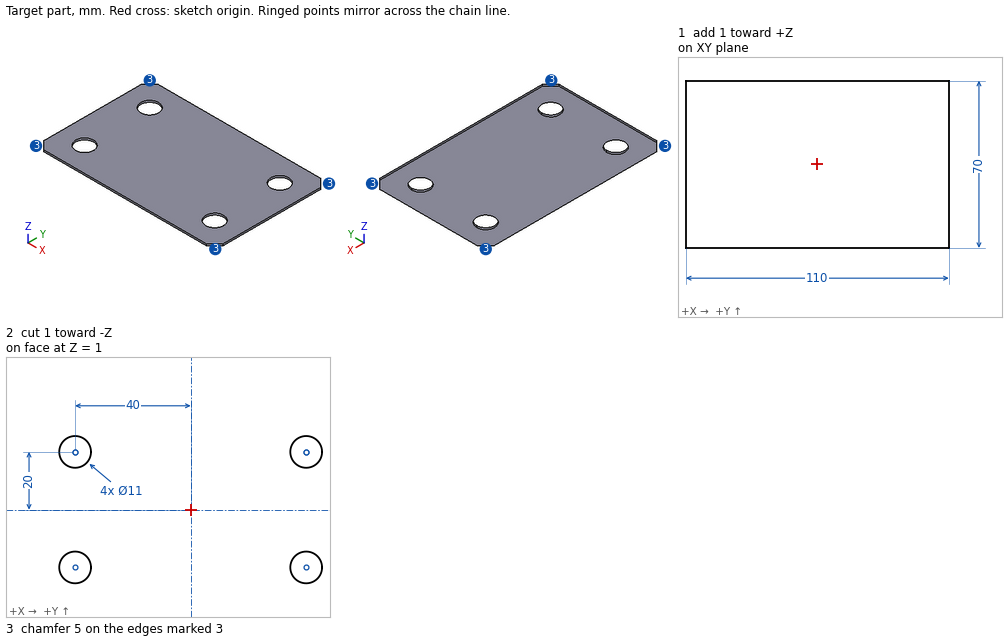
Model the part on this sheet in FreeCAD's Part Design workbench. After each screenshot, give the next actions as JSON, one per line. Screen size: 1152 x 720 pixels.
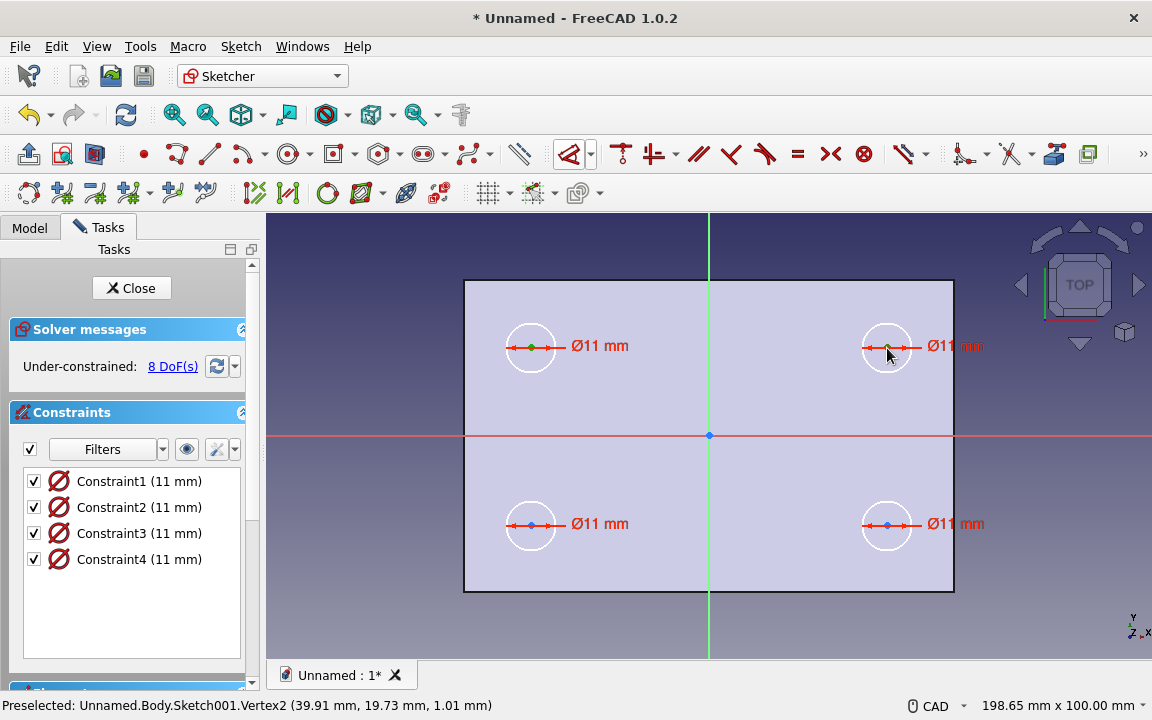
{"action": "left_click", "coordinate": [709, 603]}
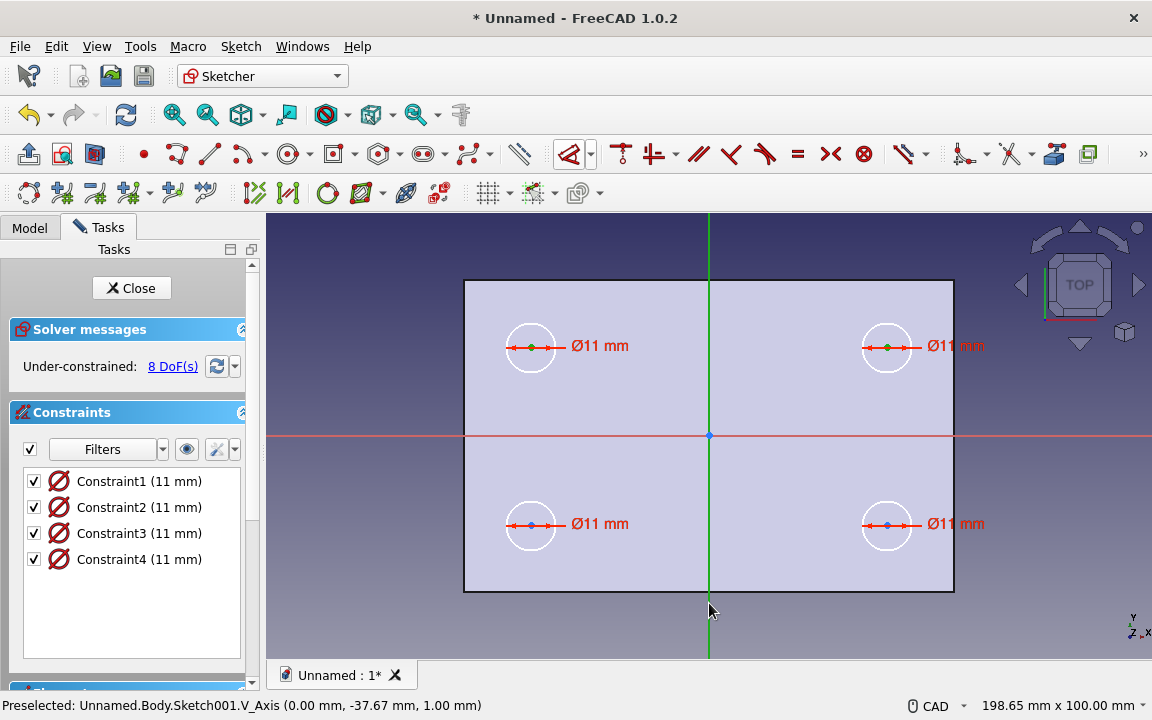
{"action": "left_click", "coordinate": [831, 154]}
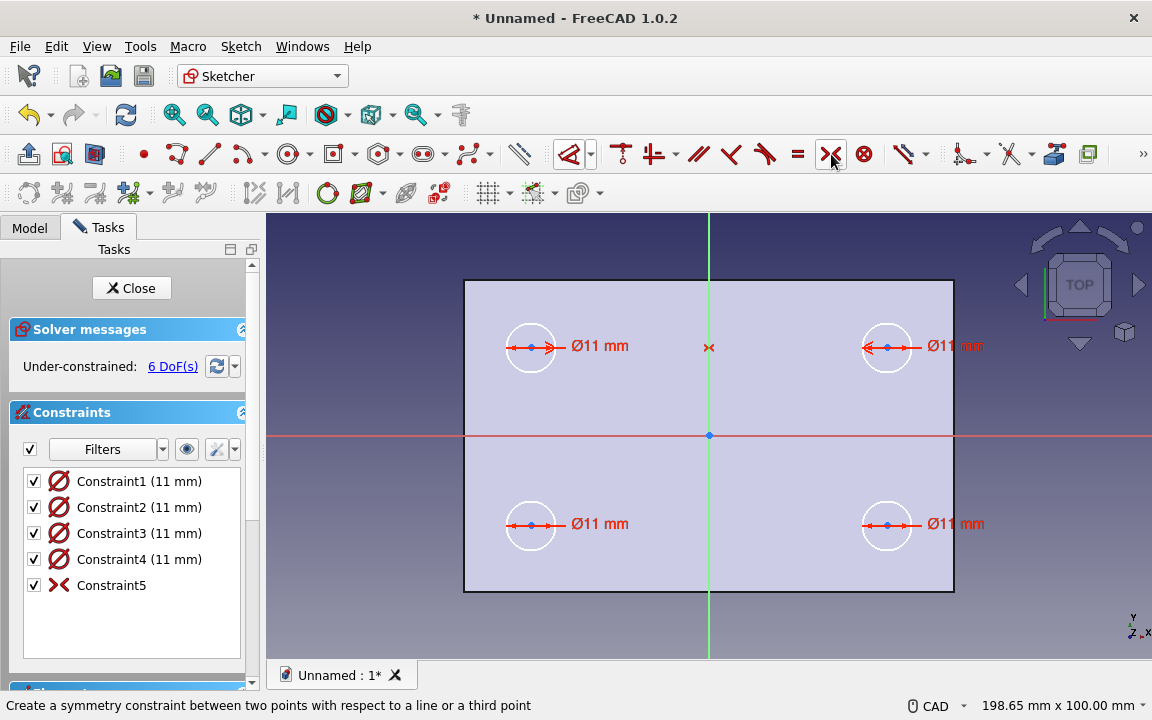
{"action": "left_click", "coordinate": [531, 348]}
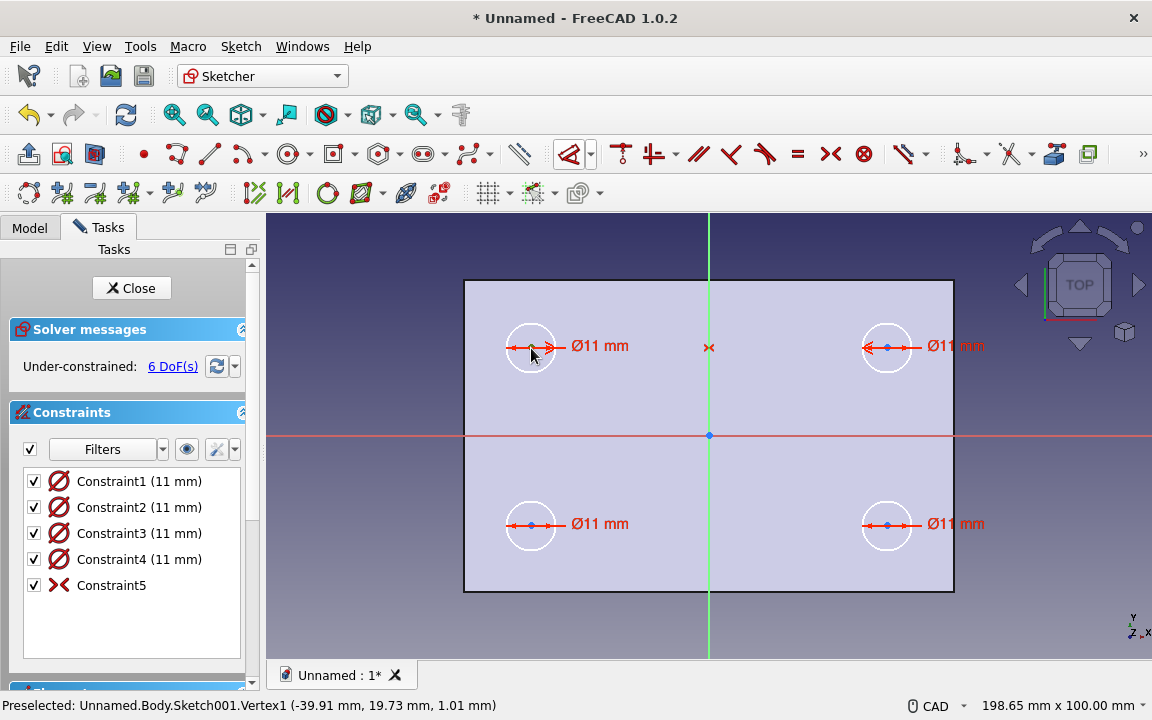
{"action": "left_click", "coordinate": [531, 526]}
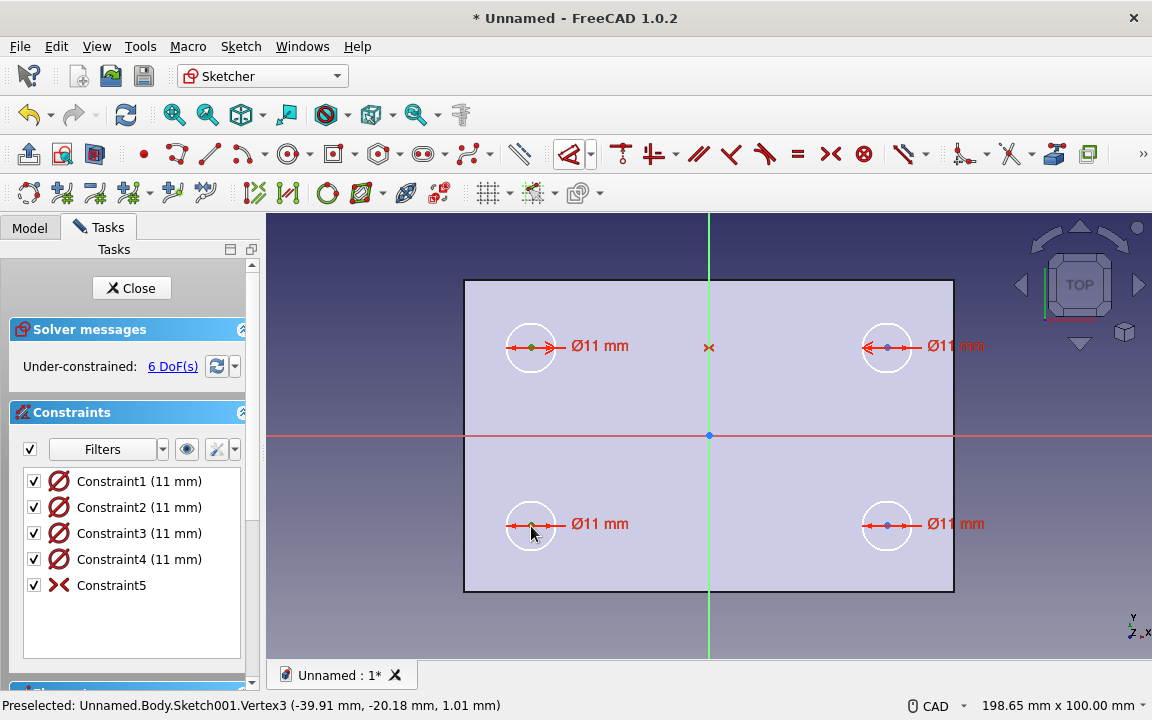
{"action": "left_click", "coordinate": [344, 436]}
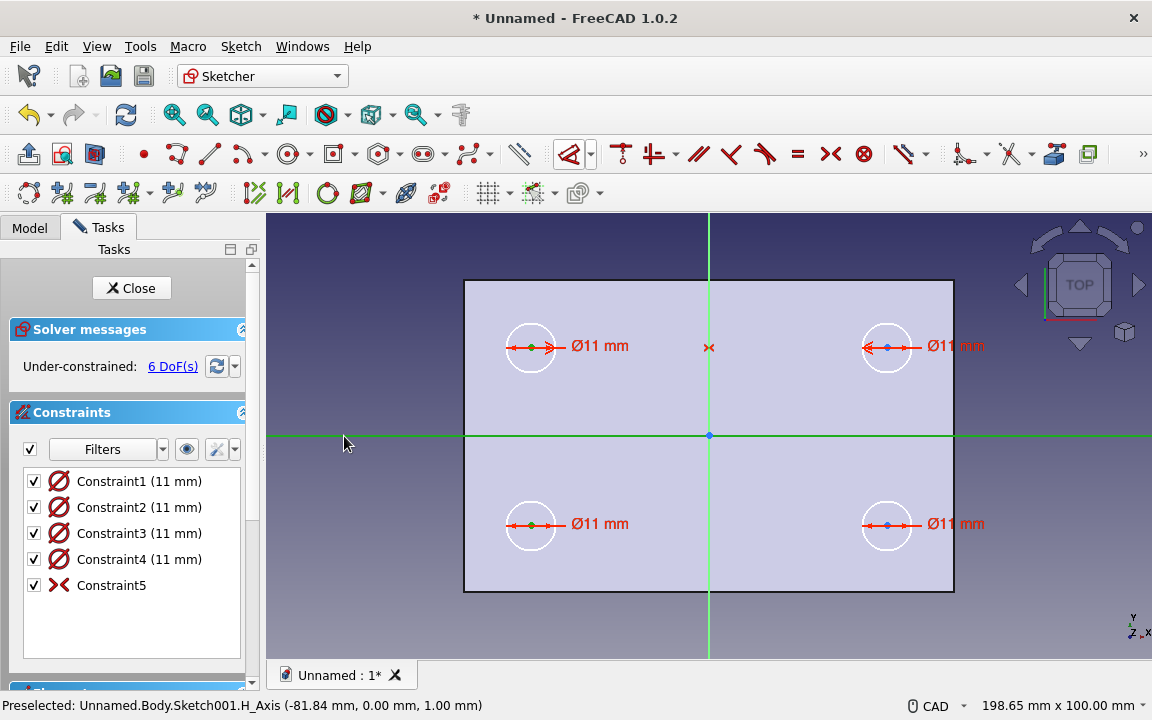
{"action": "left_click", "coordinate": [831, 154]}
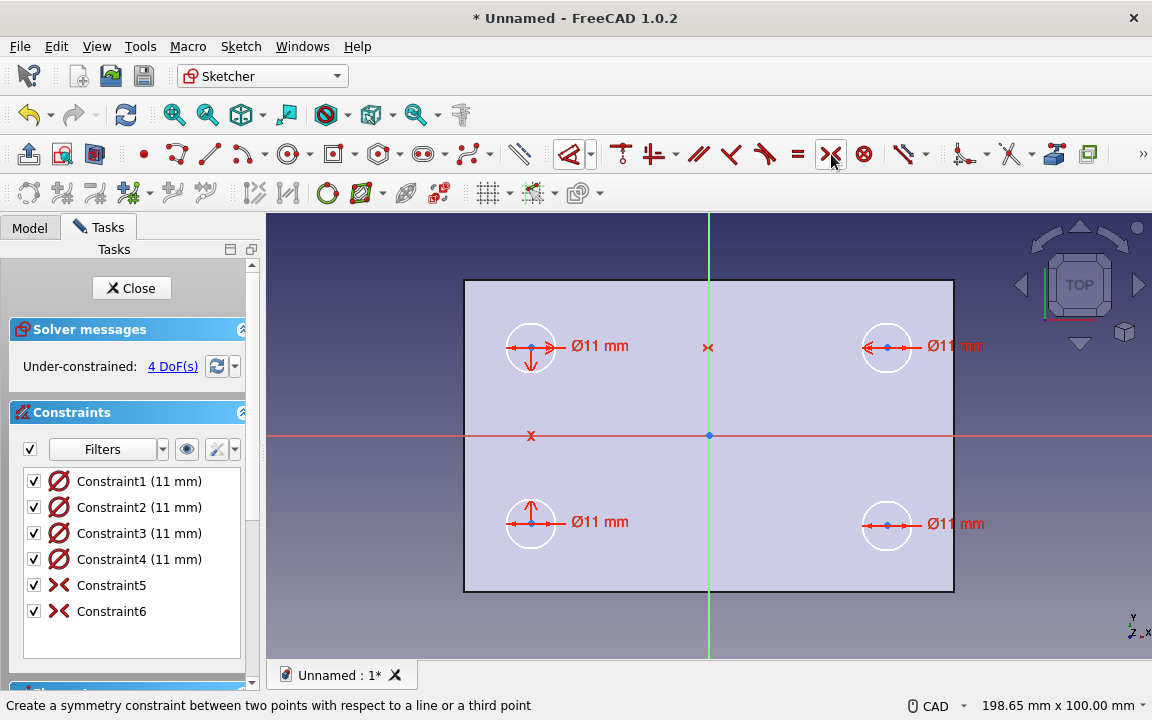
{"action": "left_click", "coordinate": [887, 348]}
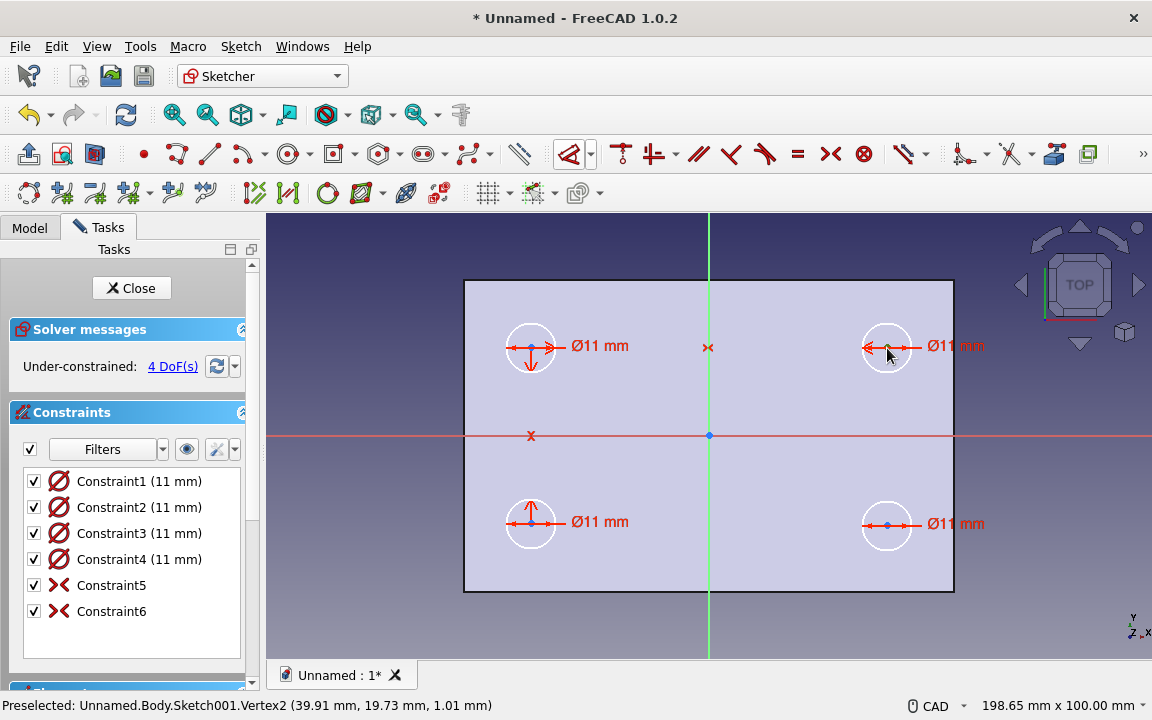
{"action": "left_click", "coordinate": [887, 526]}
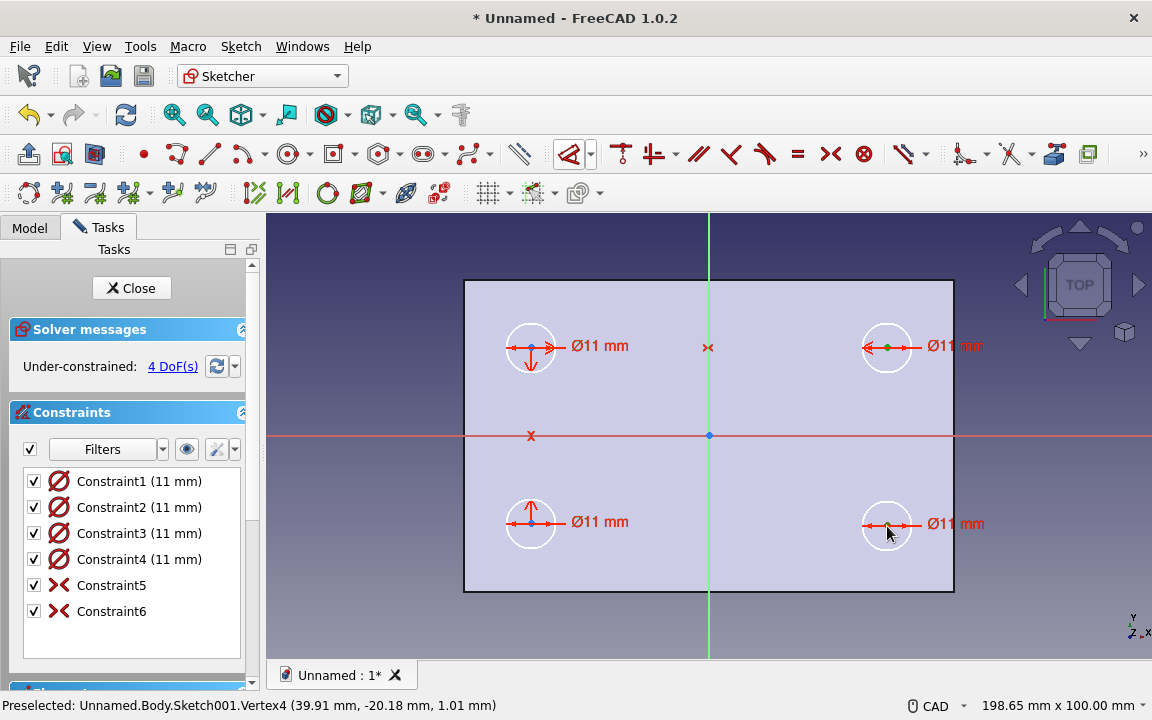
{"action": "left_click", "coordinate": [344, 436]}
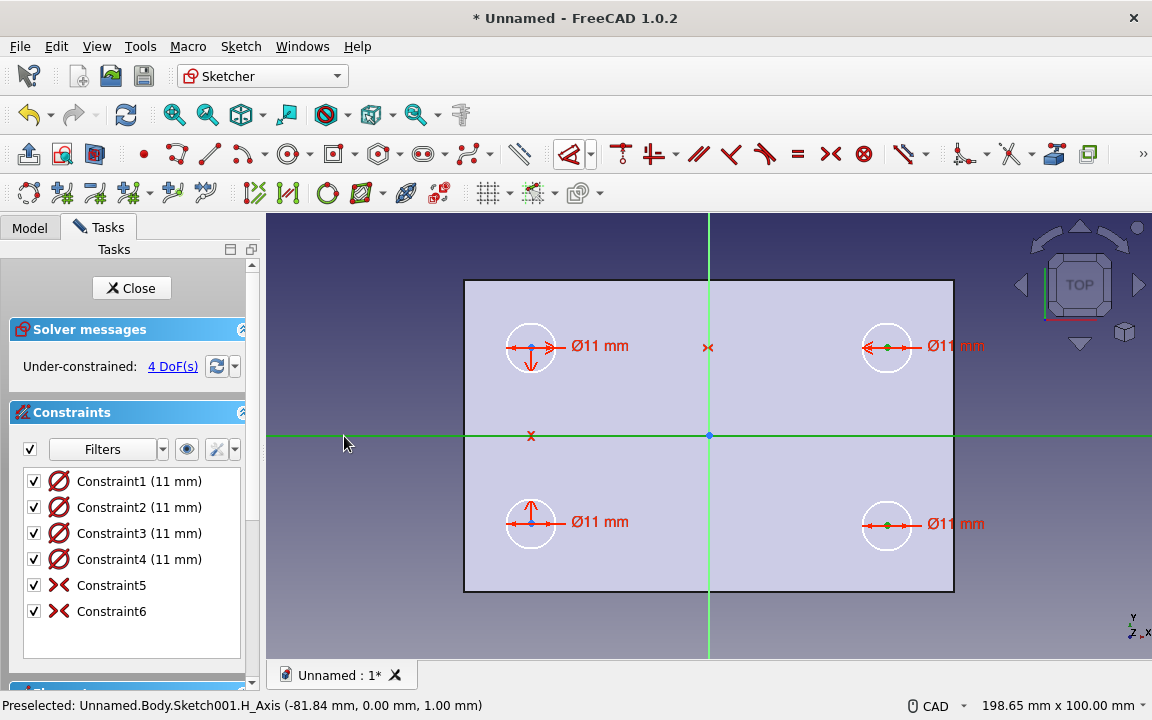
{"action": "left_click", "coordinate": [831, 154]}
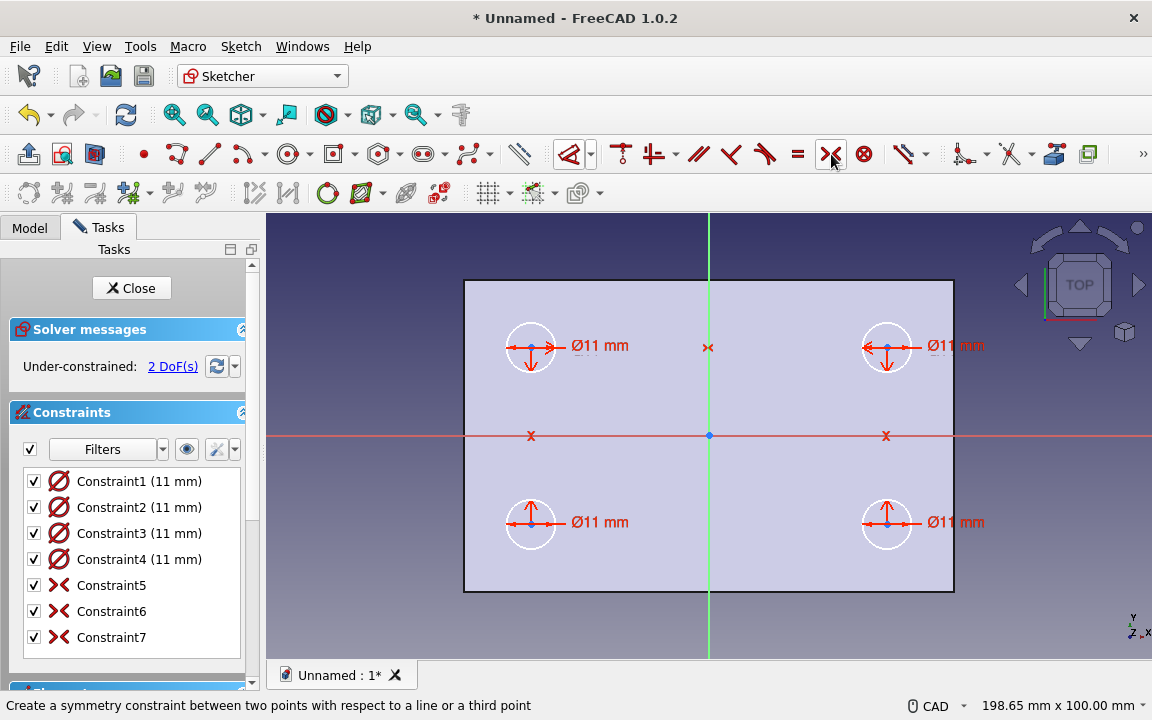
{"action": "left_click", "coordinate": [568, 154]}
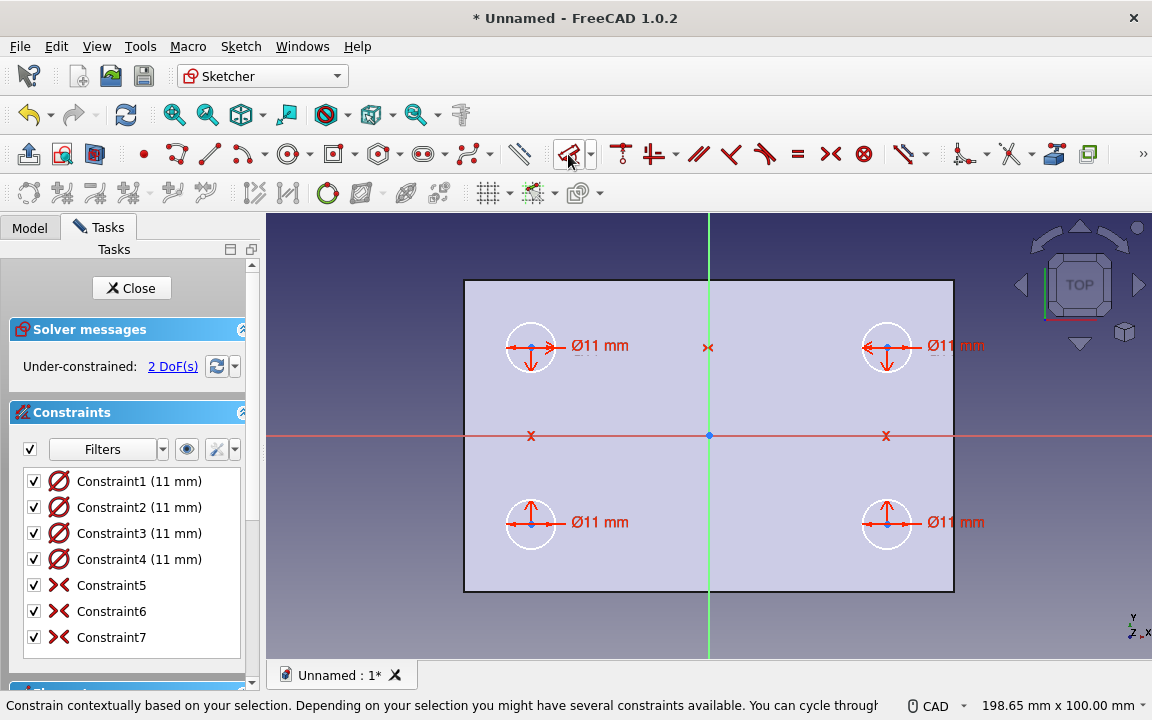
{"action": "left_click", "coordinate": [531, 348]}
{"action": "left_click", "coordinate": [620, 314]}